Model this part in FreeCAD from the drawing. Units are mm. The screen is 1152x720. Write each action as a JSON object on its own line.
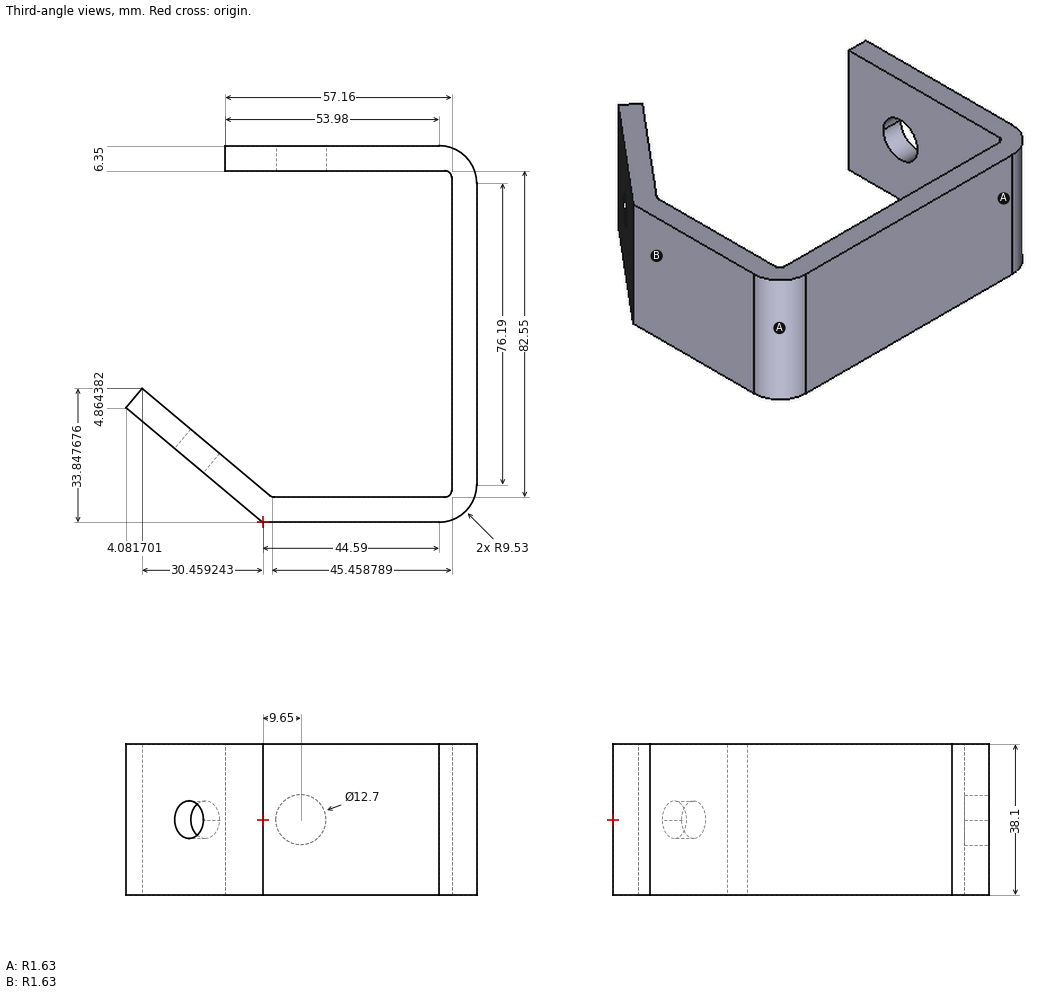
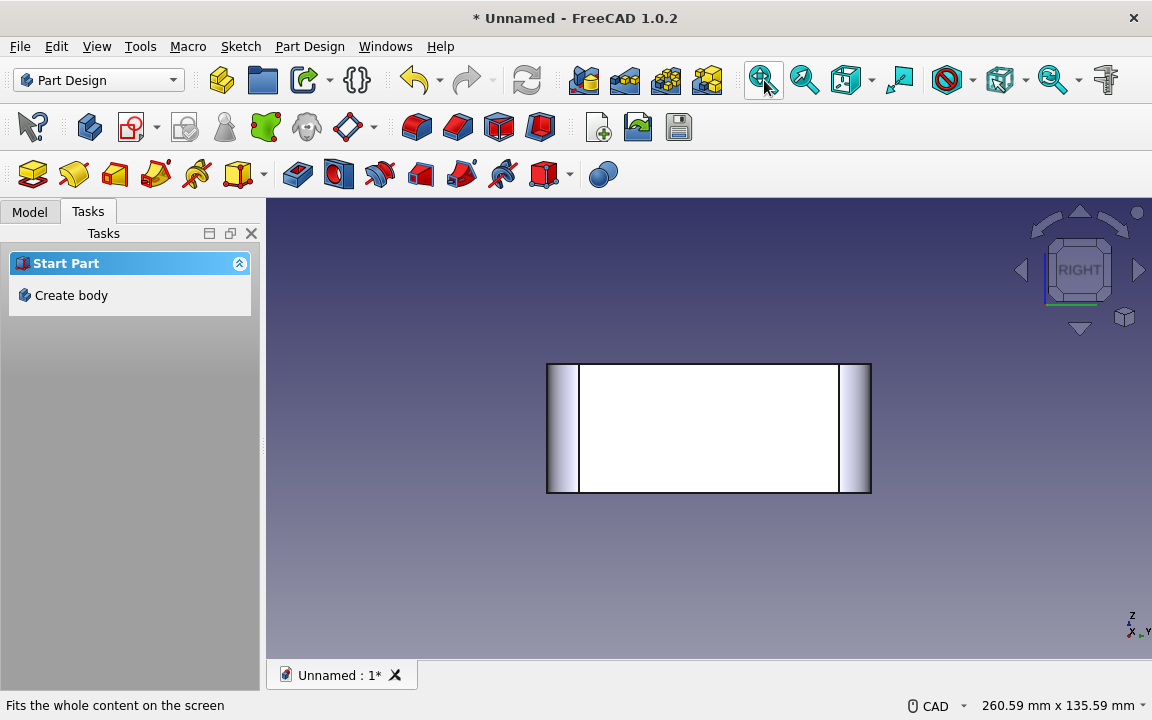
{"action": "key", "text": "5"}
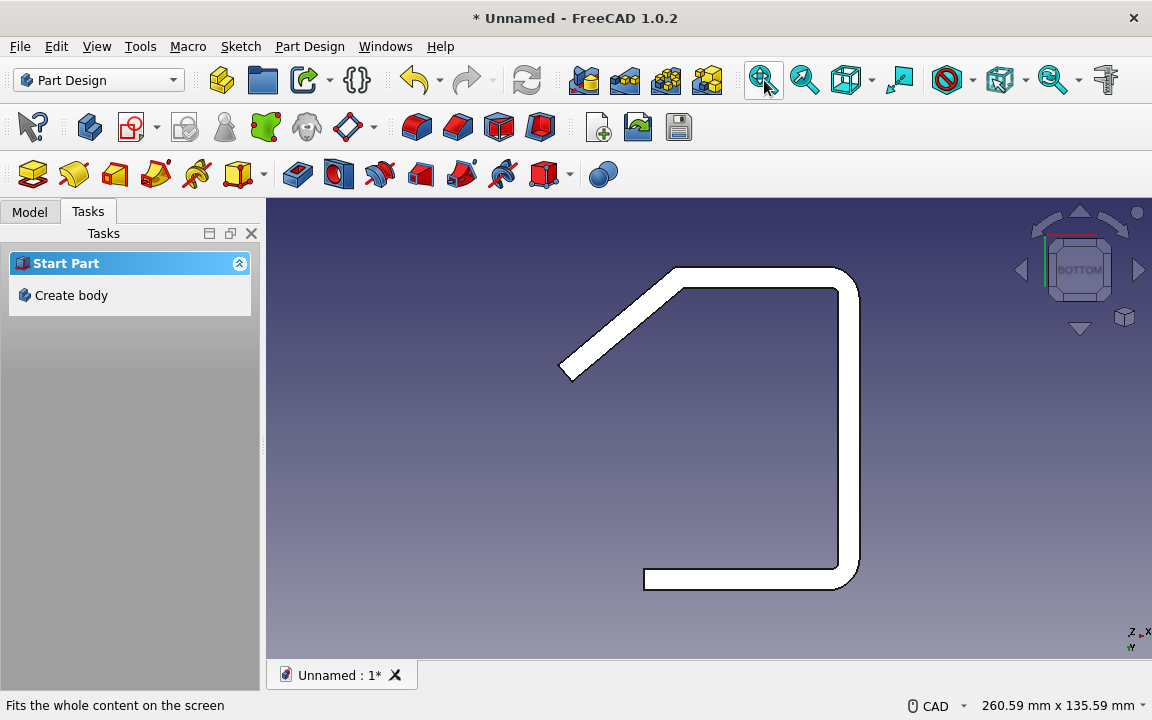
{"action": "key", "text": "4"}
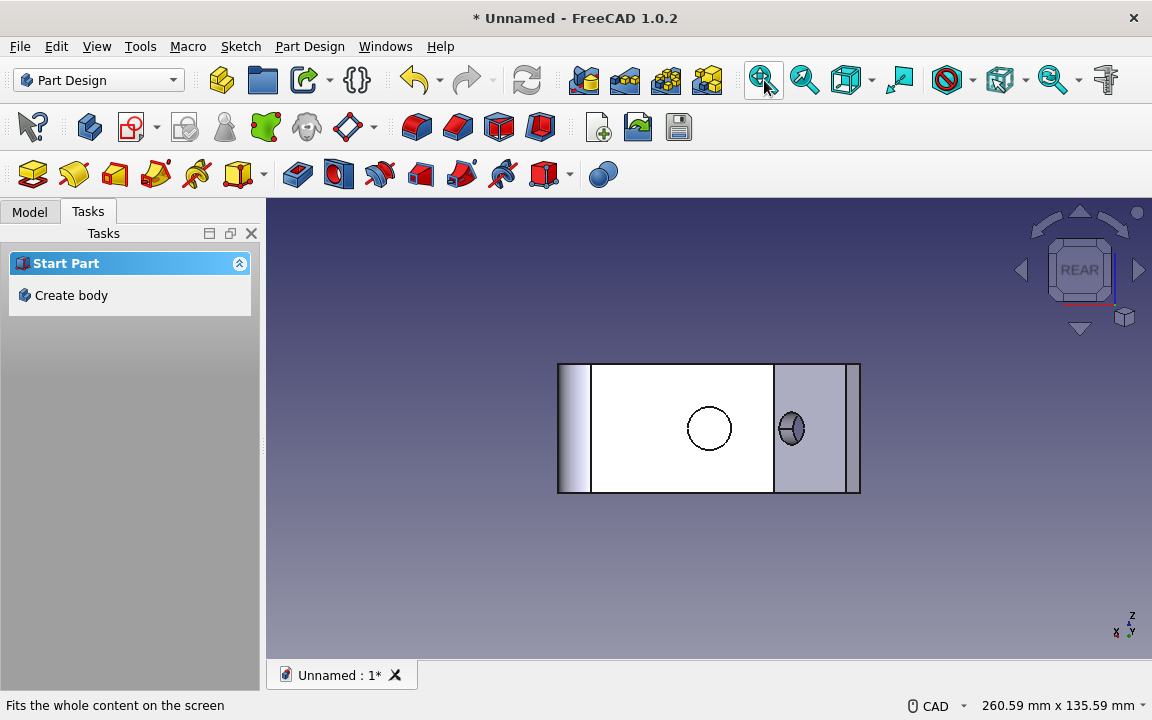
{"action": "key", "text": "v f"}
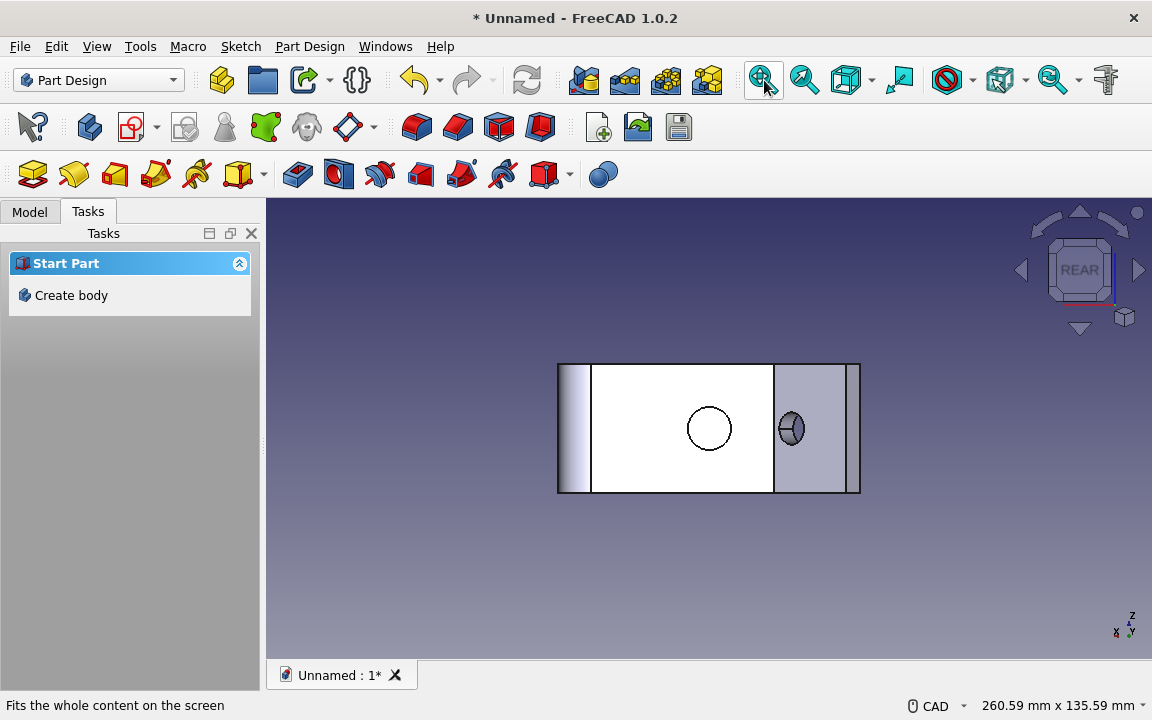
{"action": "key", "text": "6"}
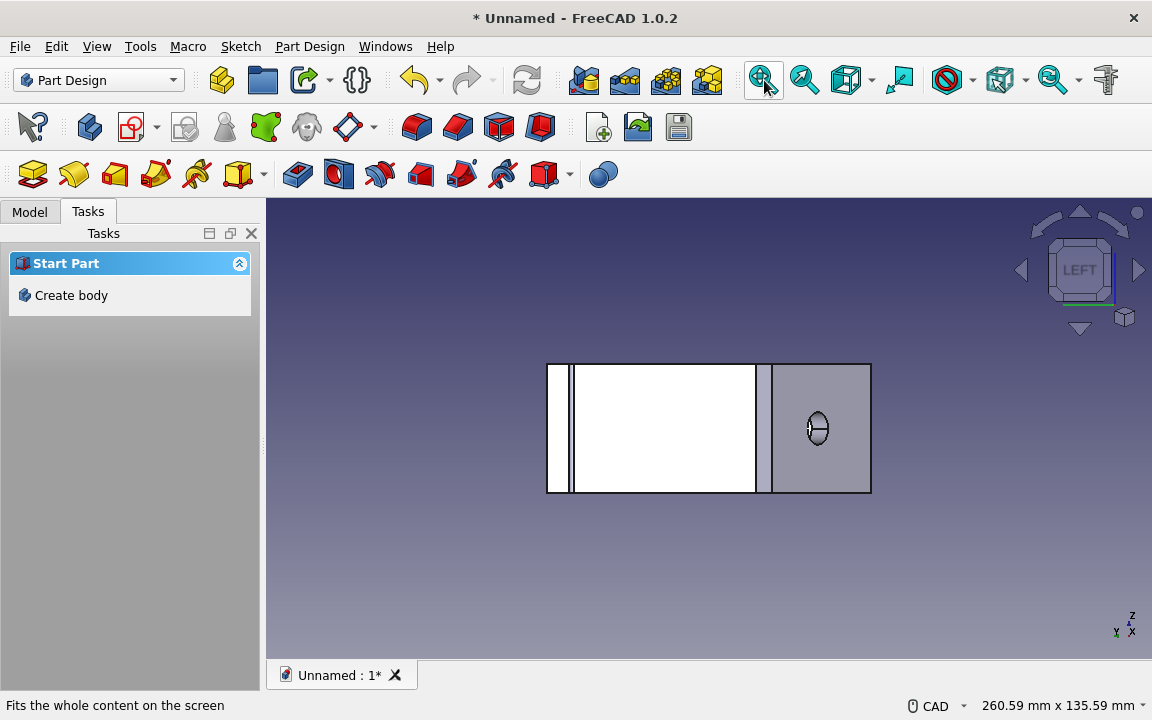
{"action": "left_click", "coordinate": [764, 80]}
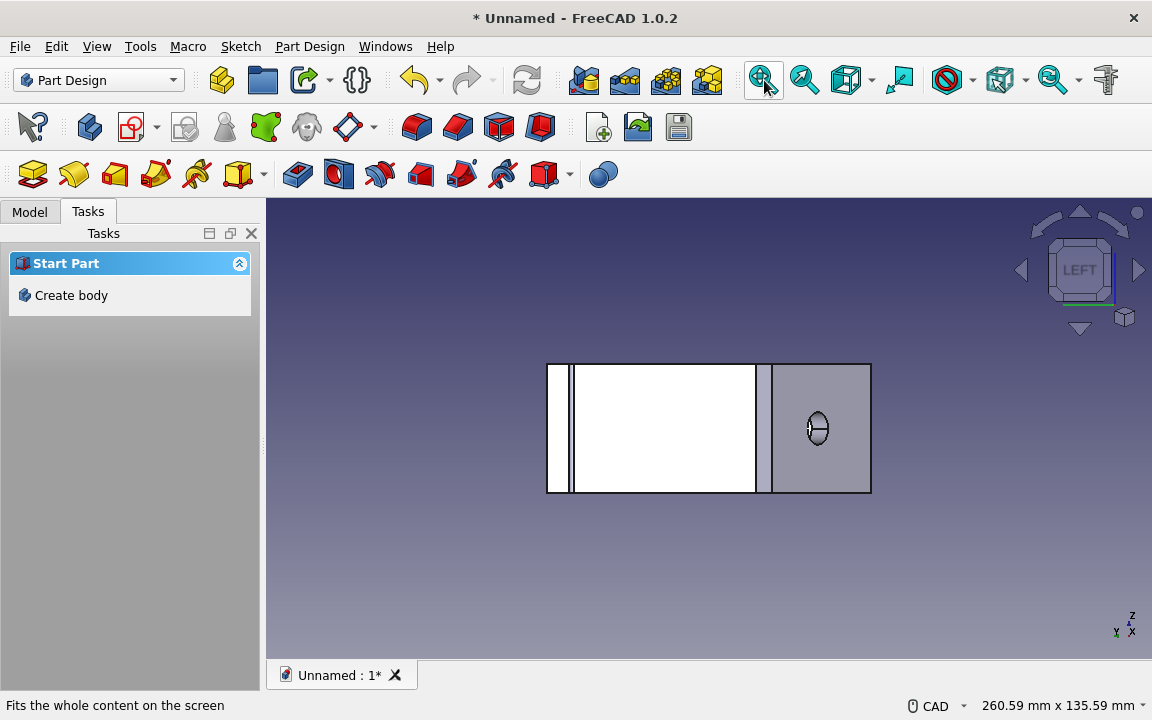
{"action": "key", "text": "v 3"}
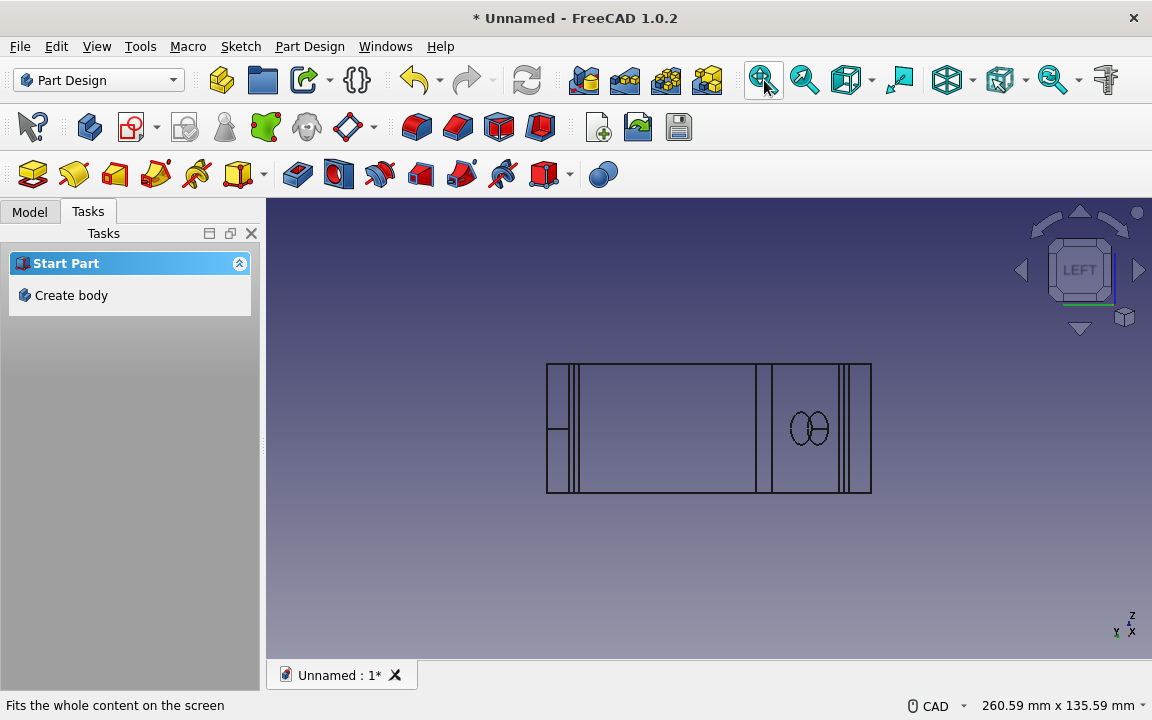
{"action": "key", "text": "0"}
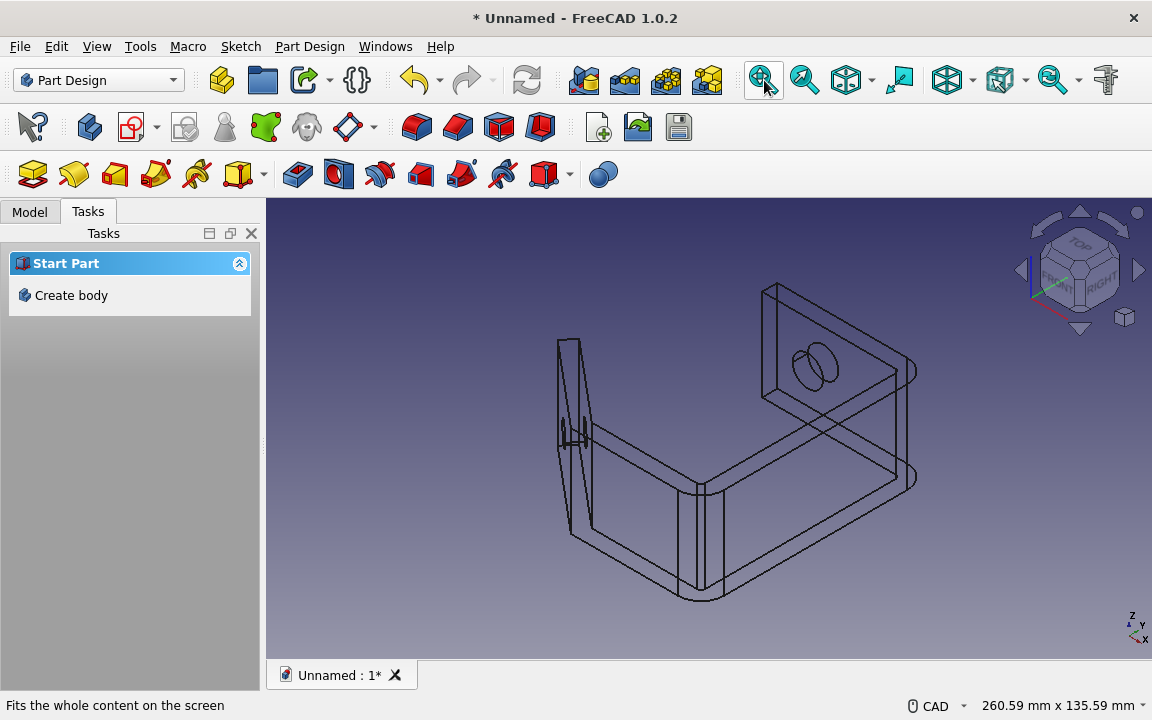
{"action": "left_click", "coordinate": [592, 474]}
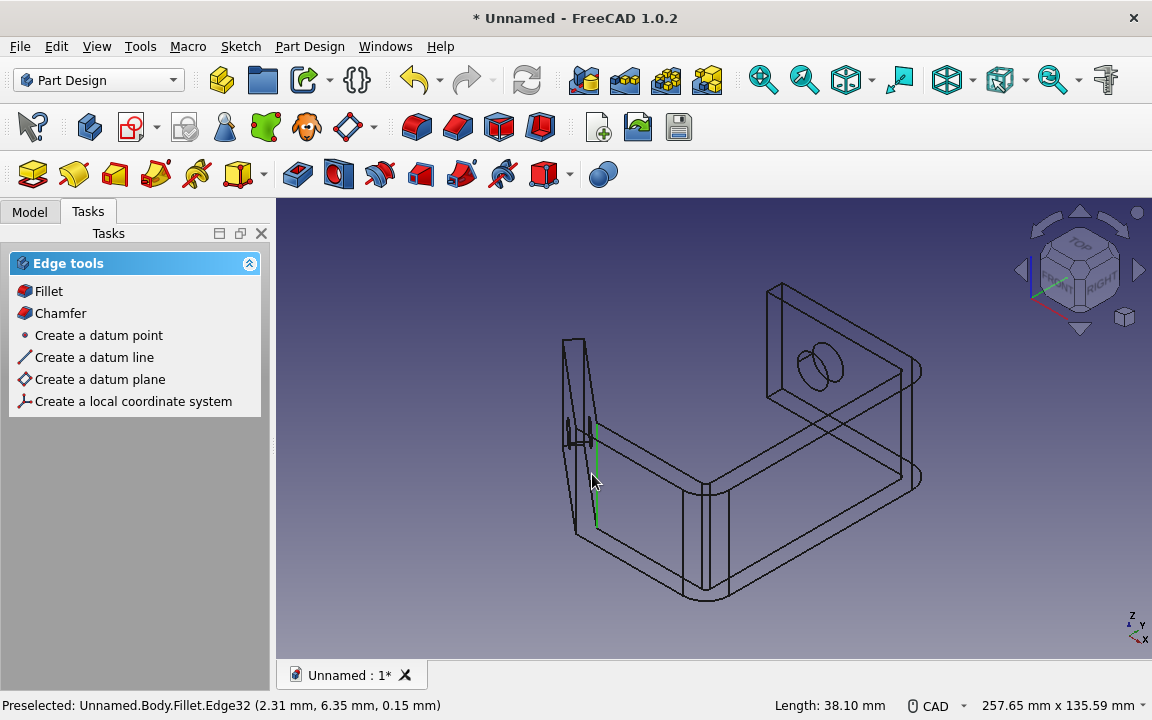
{"action": "key", "text": "v 1"}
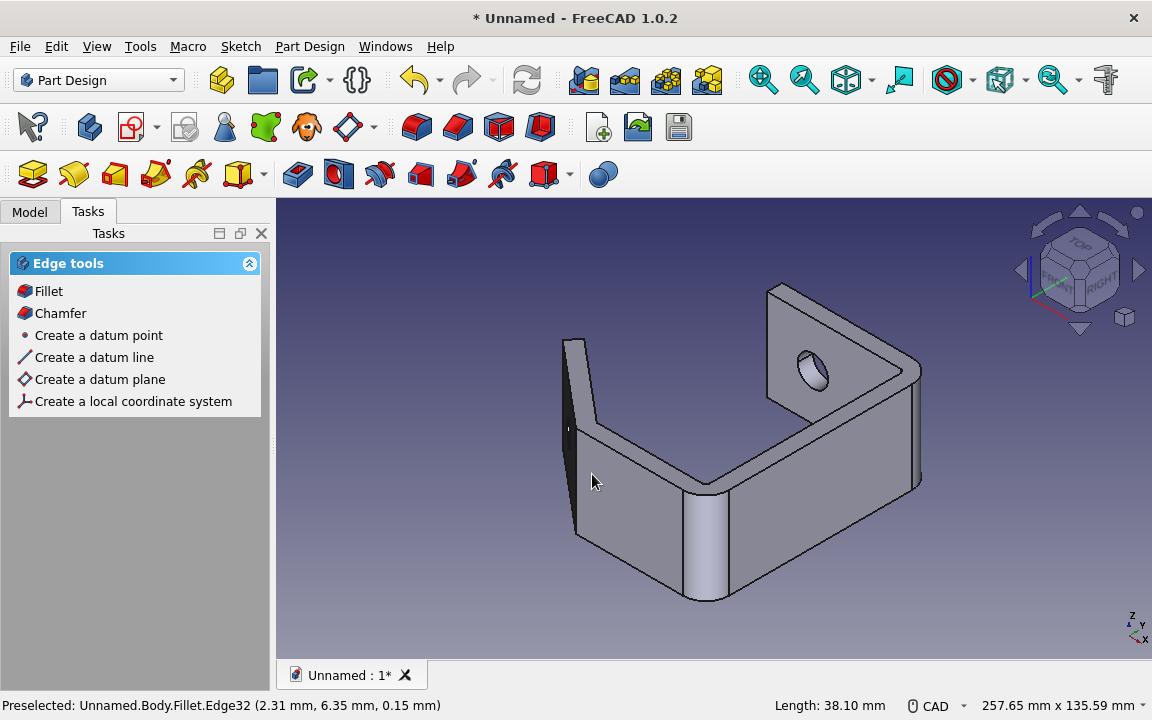
{"action": "left_click", "coordinate": [417, 128]}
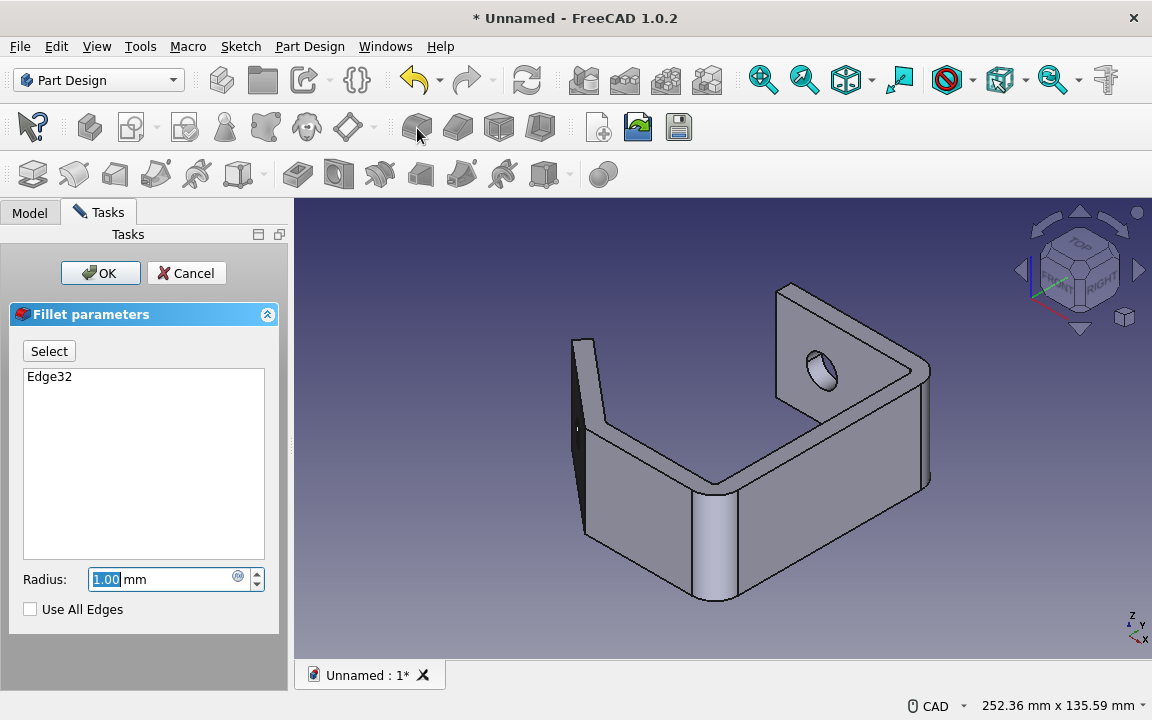
{"action": "type", "text": "1.63"}
{"action": "key", "text": "Tab"}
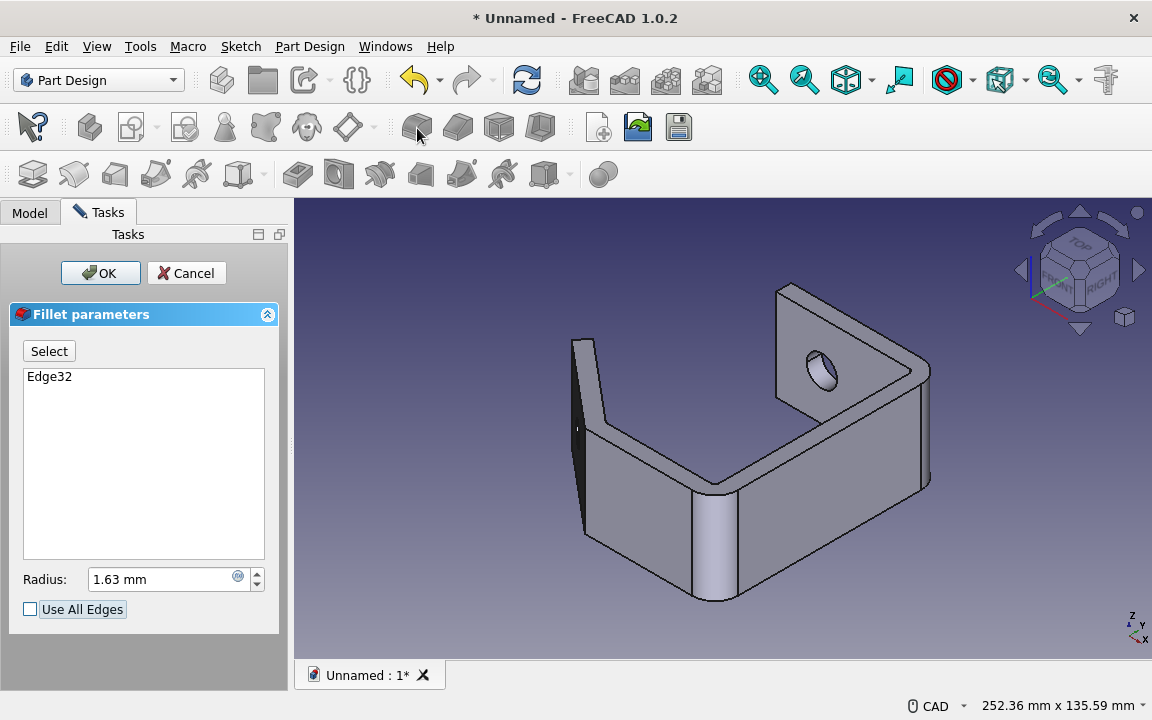
{"action": "left_click", "coordinate": [101, 273]}